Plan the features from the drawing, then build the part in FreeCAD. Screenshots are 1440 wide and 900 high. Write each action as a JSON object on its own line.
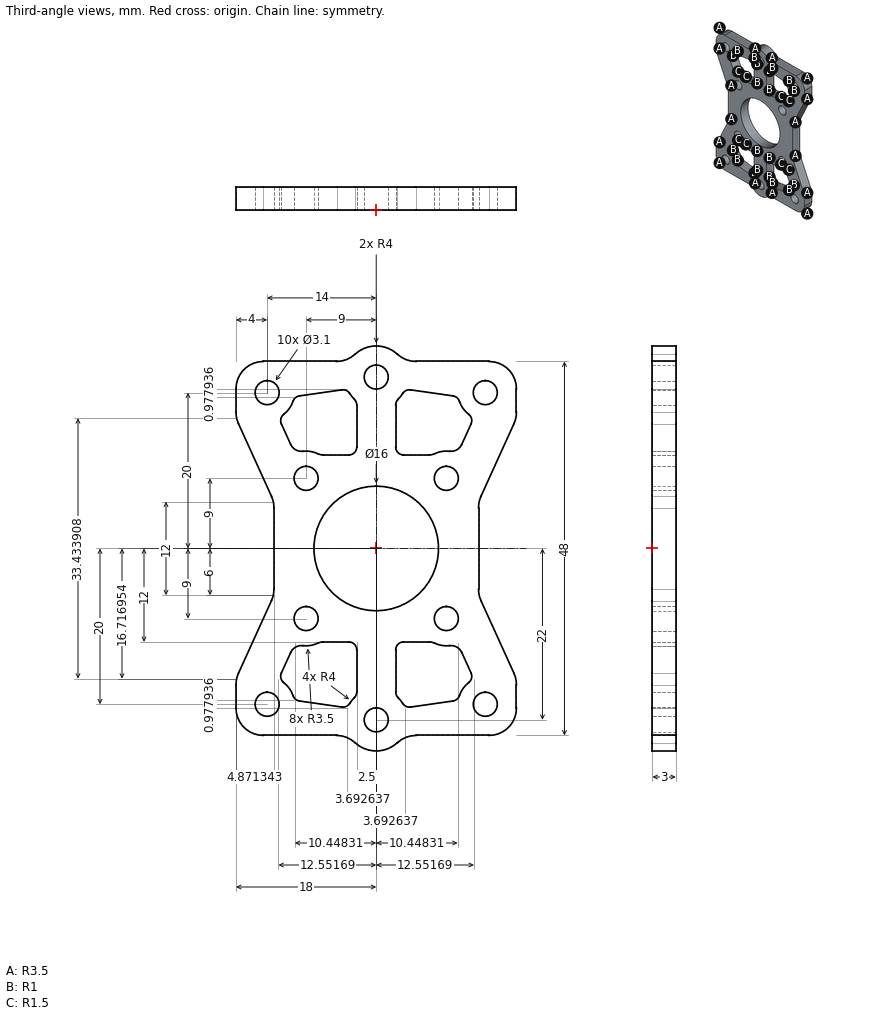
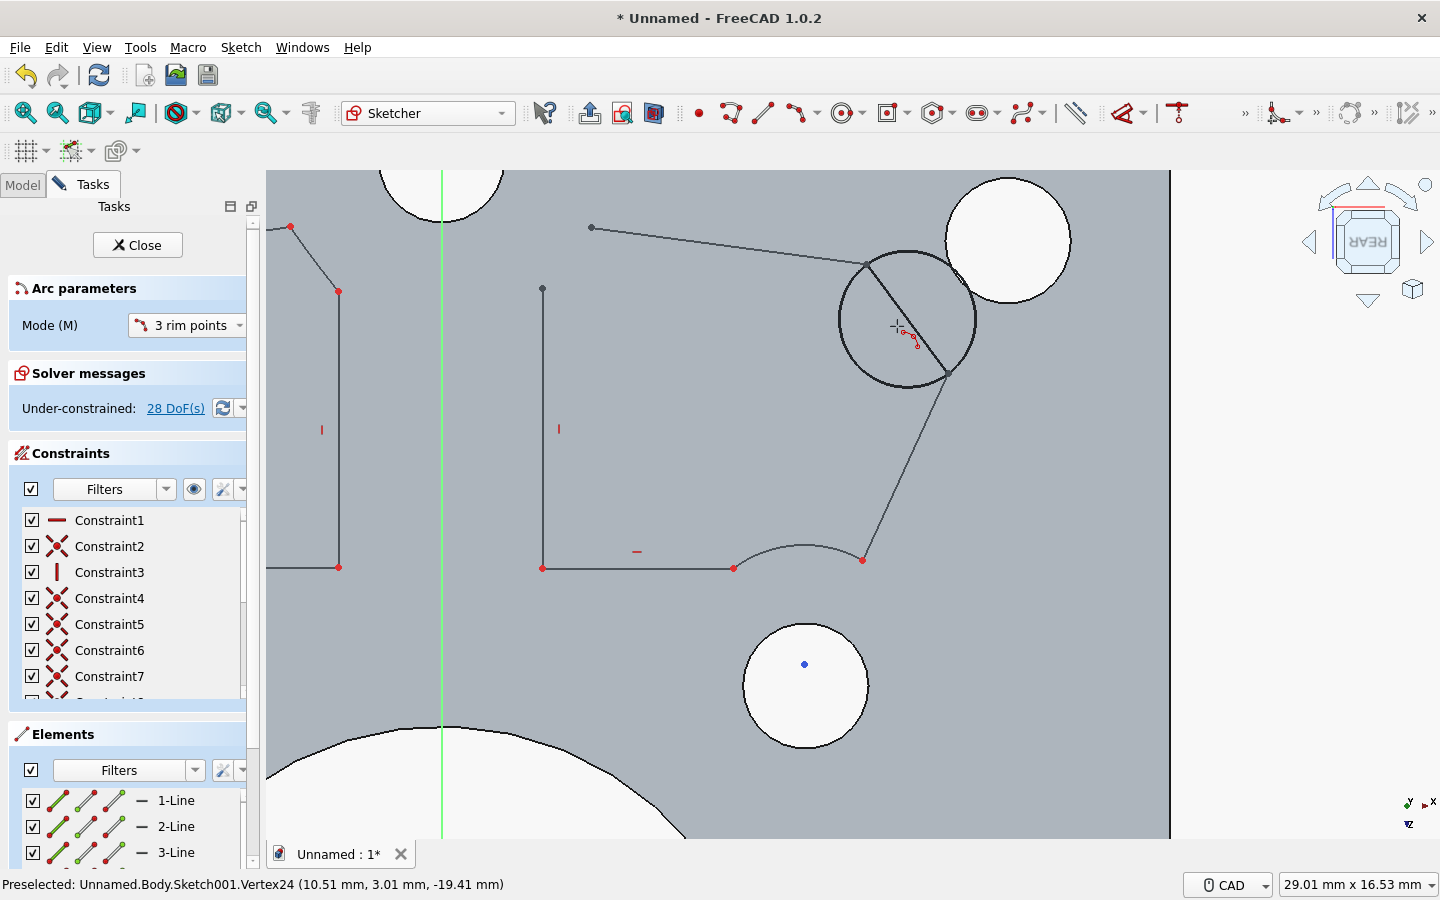
{"action": "left_click", "coordinate": [895, 326]}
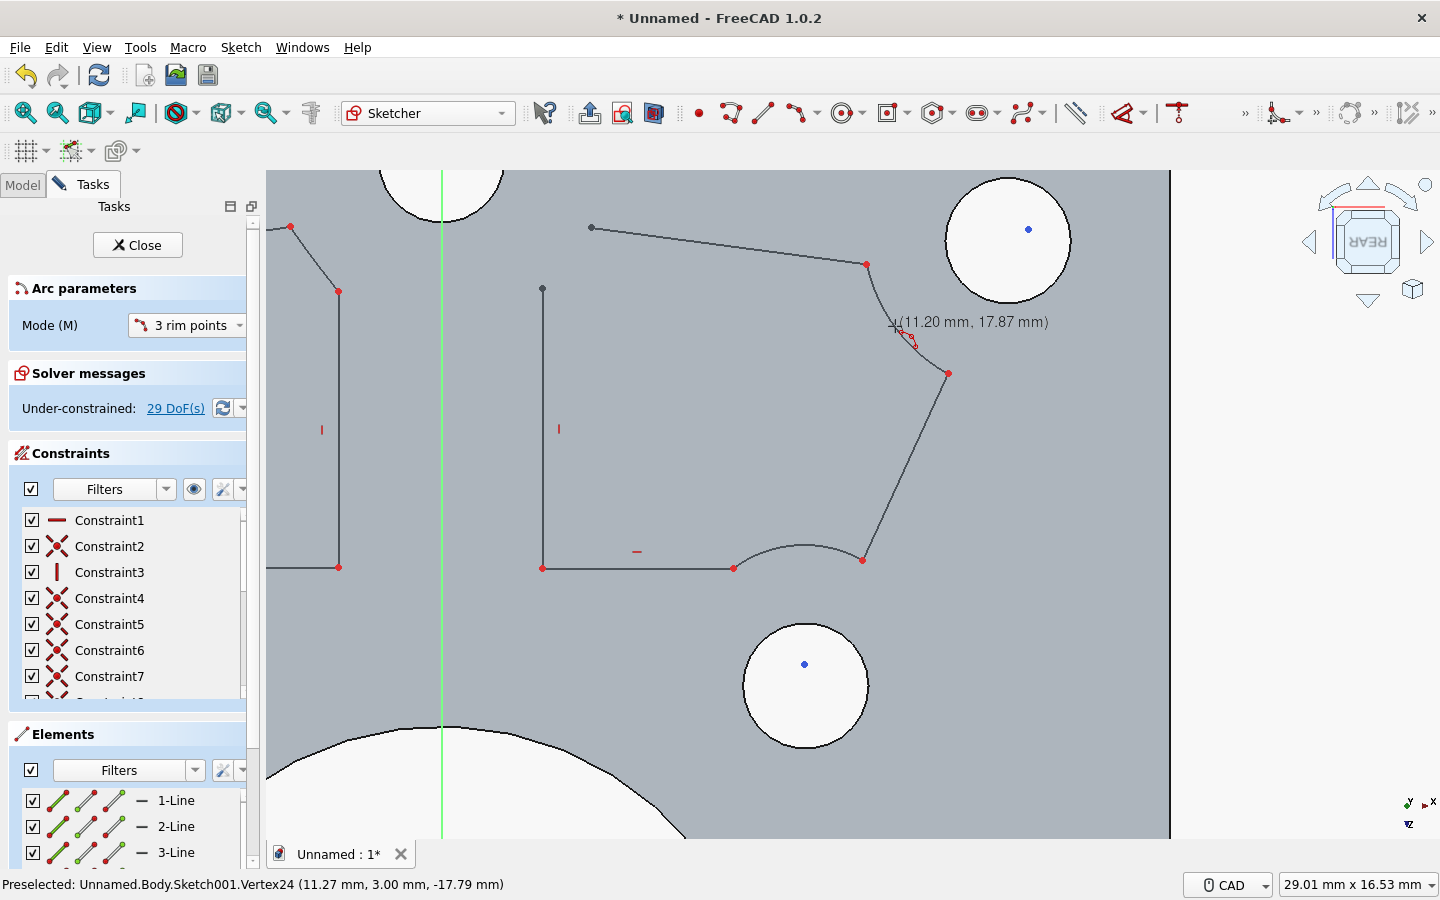
{"action": "scroll", "coordinate": [897, 326], "scroll_direction": "down", "scroll_amount": 7}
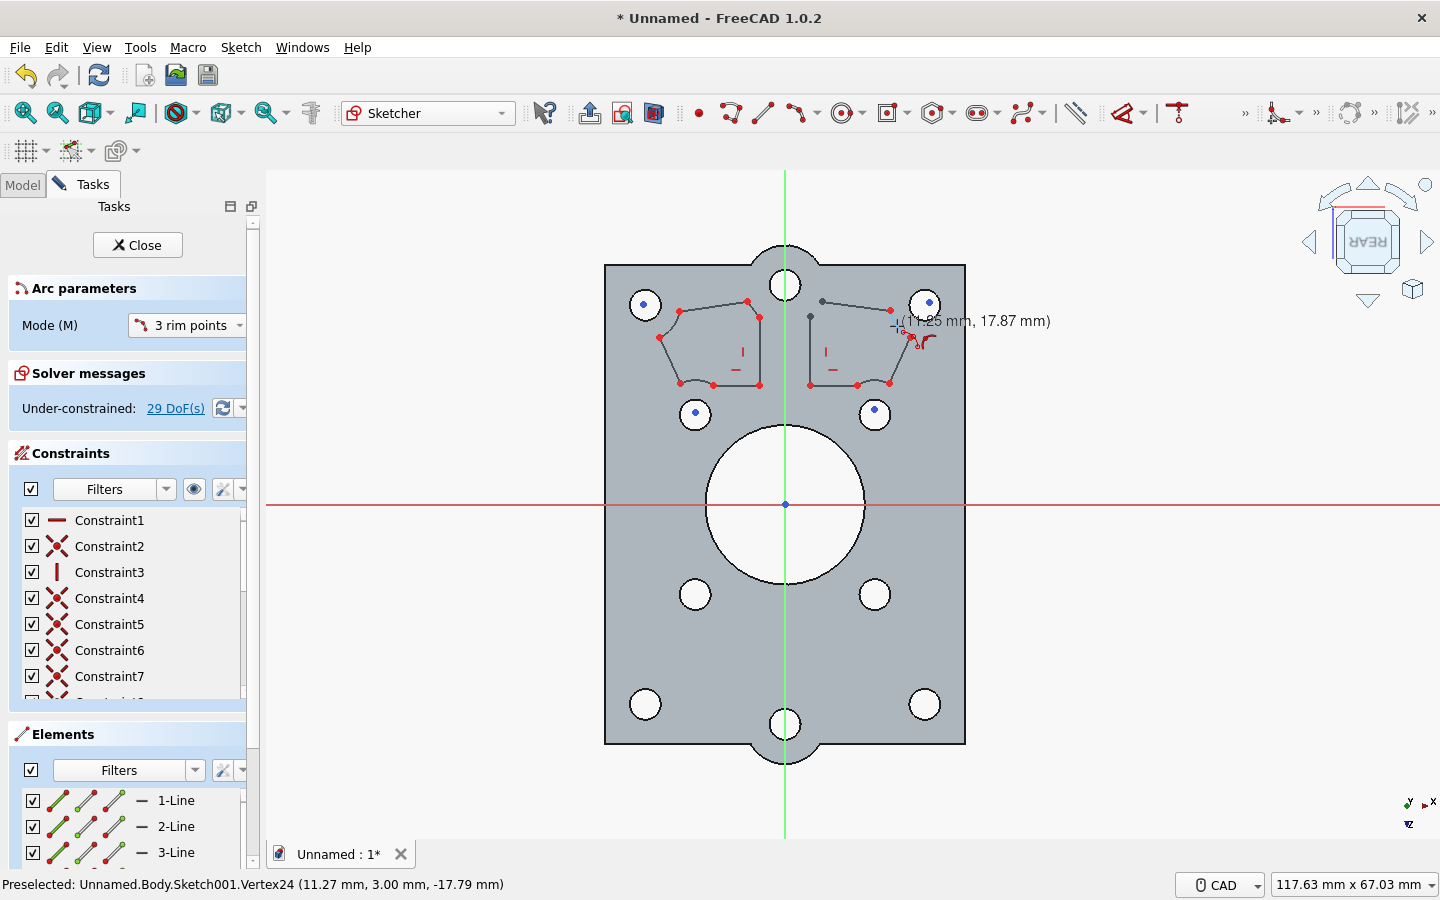
{"action": "left_click", "coordinate": [822, 302]}
{"action": "left_click", "coordinate": [810, 317]}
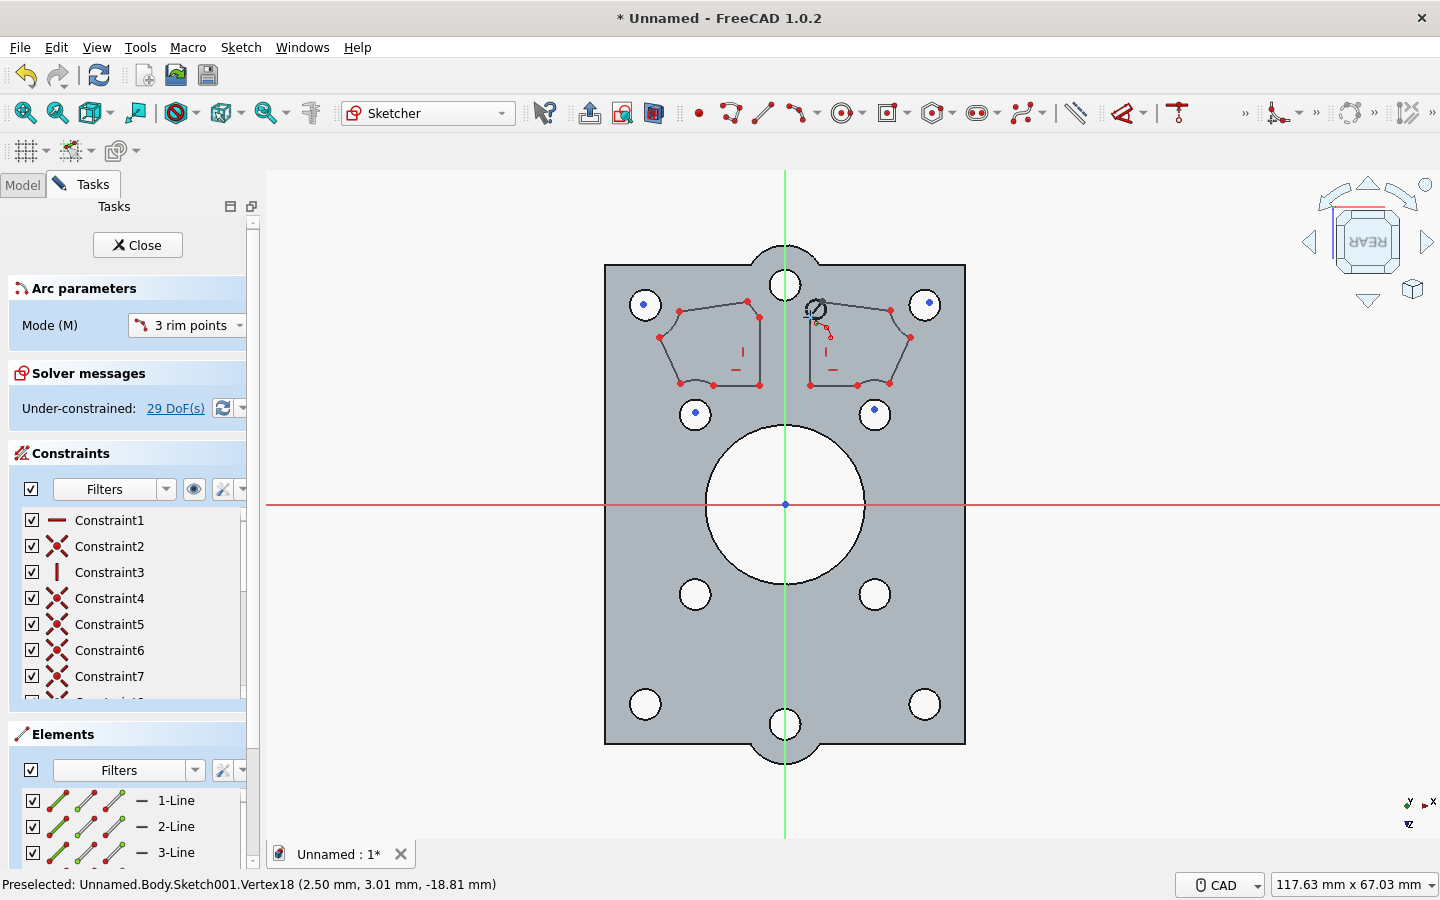
{"action": "scroll", "coordinate": [817, 309], "scroll_direction": "up", "scroll_amount": 13}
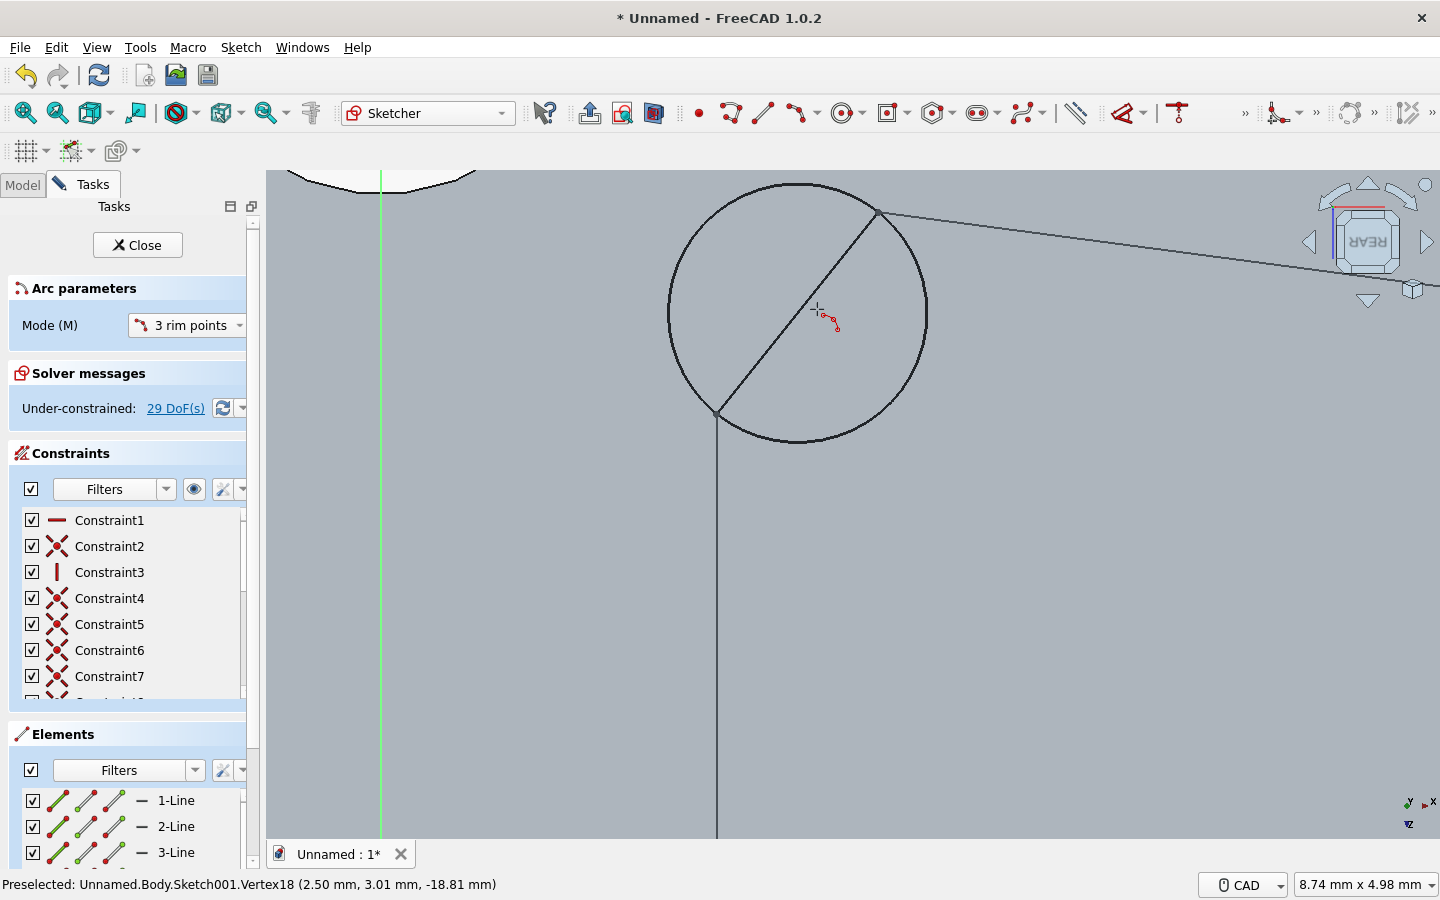
{"action": "left_click", "coordinate": [811, 309]}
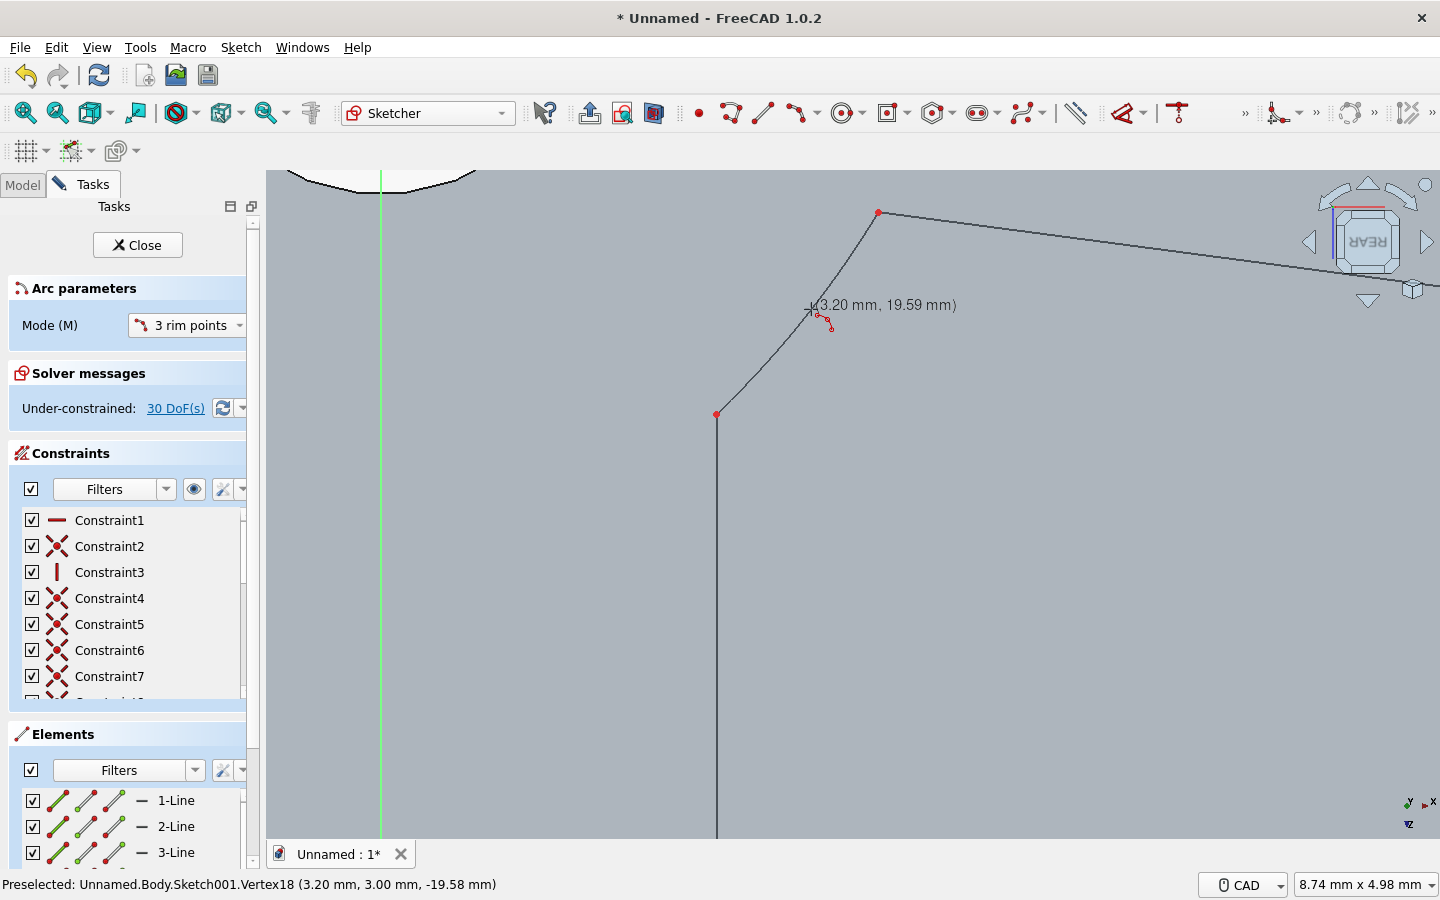
{"action": "left_click", "coordinate": [732, 114]}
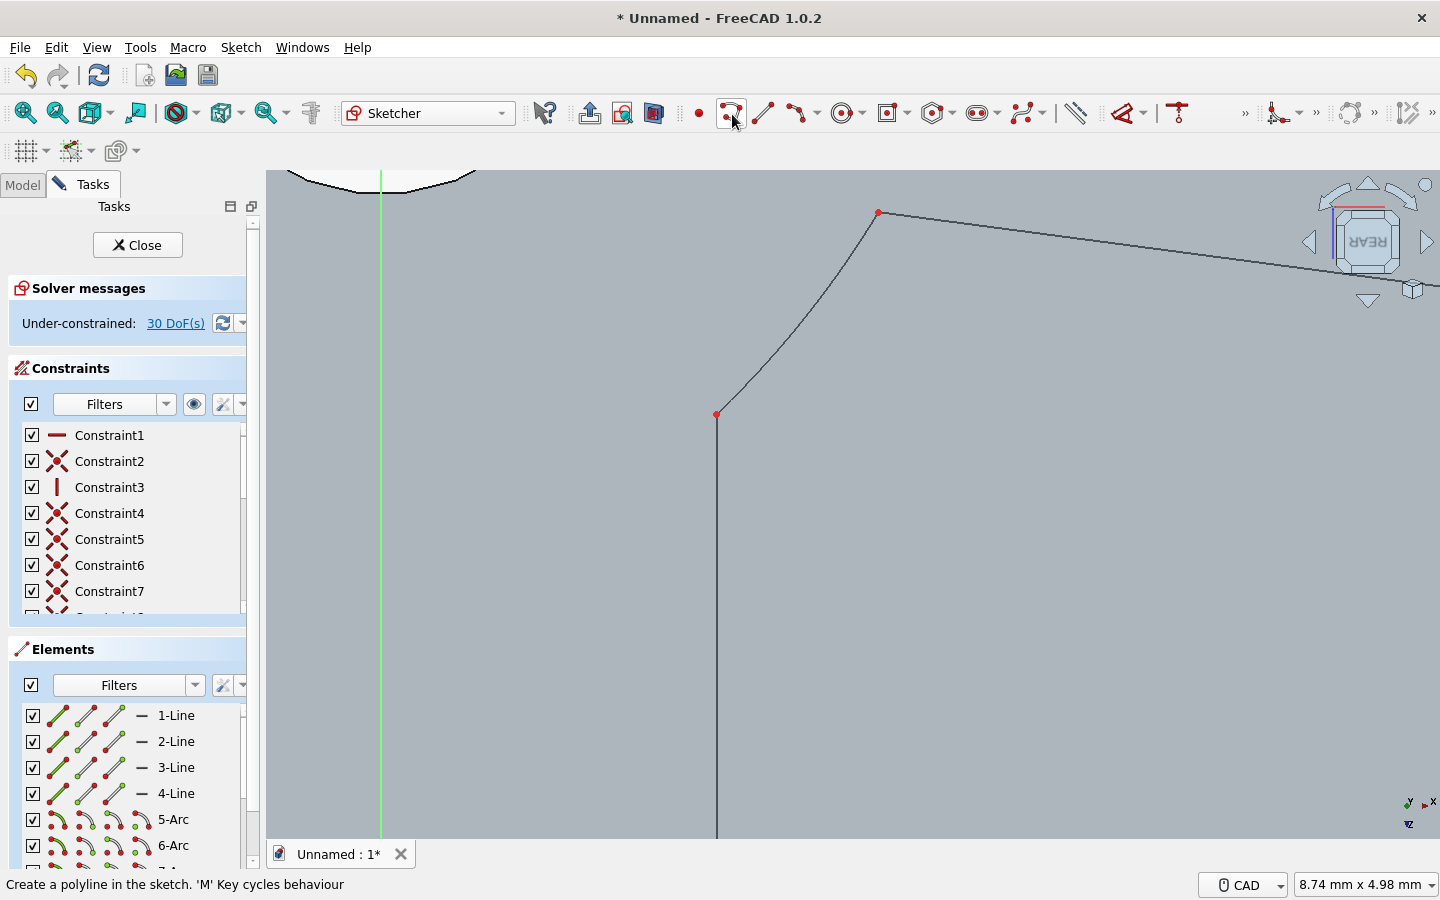
{"action": "scroll", "coordinate": [817, 309], "scroll_direction": "down", "scroll_amount": 13}